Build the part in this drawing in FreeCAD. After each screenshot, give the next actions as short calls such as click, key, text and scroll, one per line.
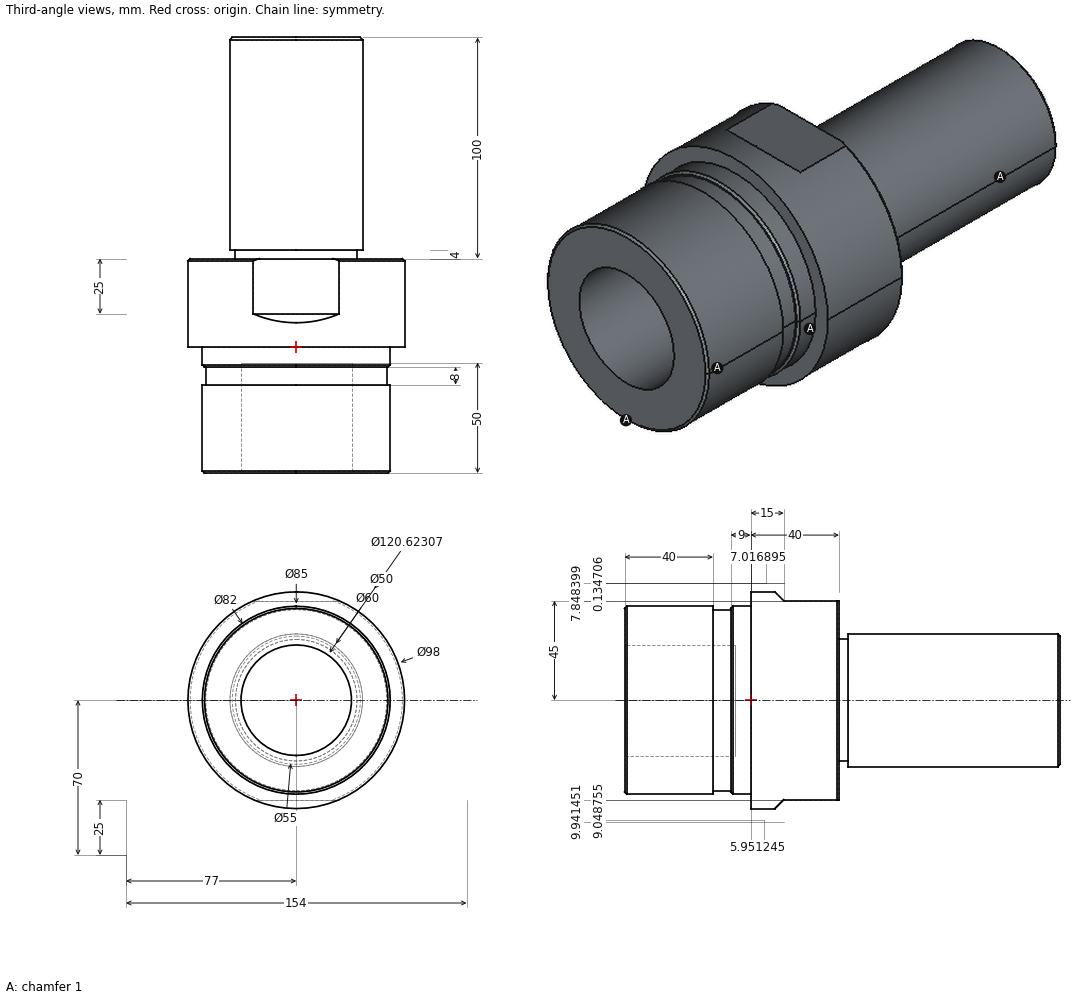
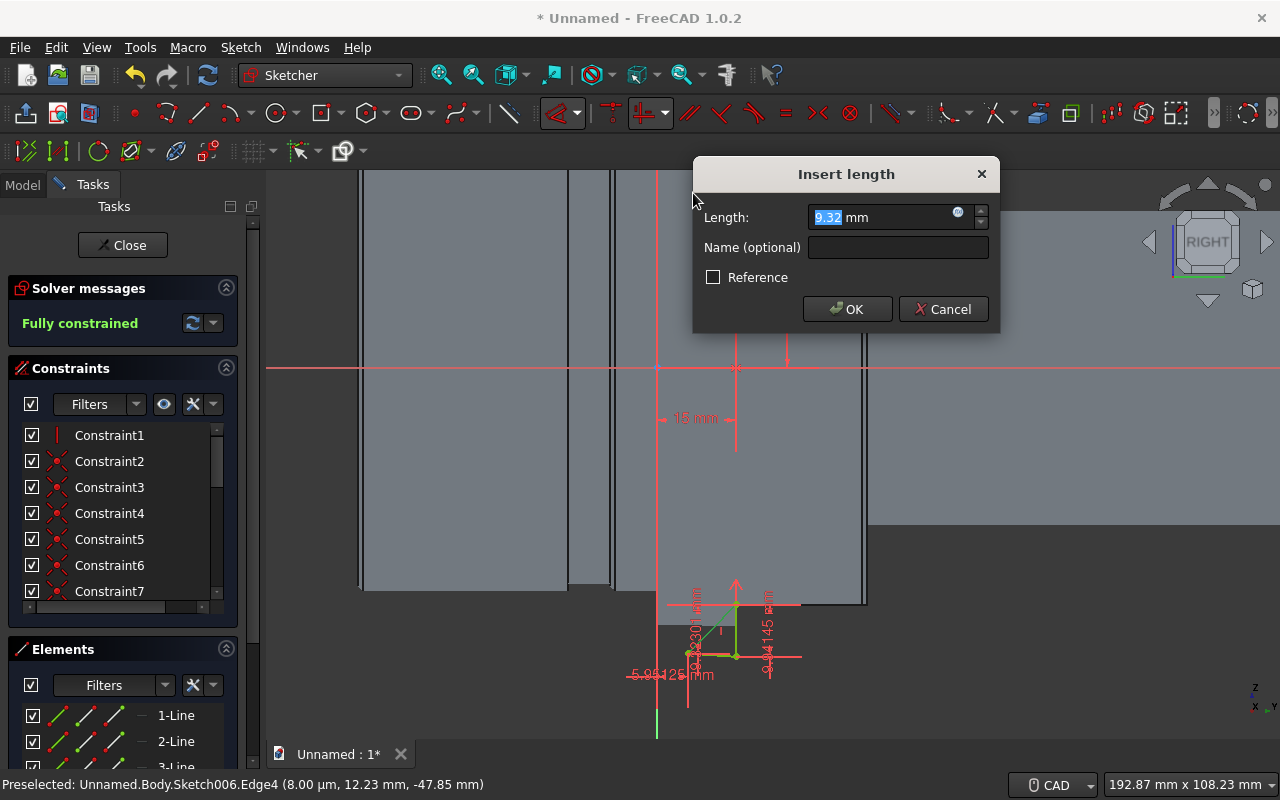
text(9.048755)
key(Return)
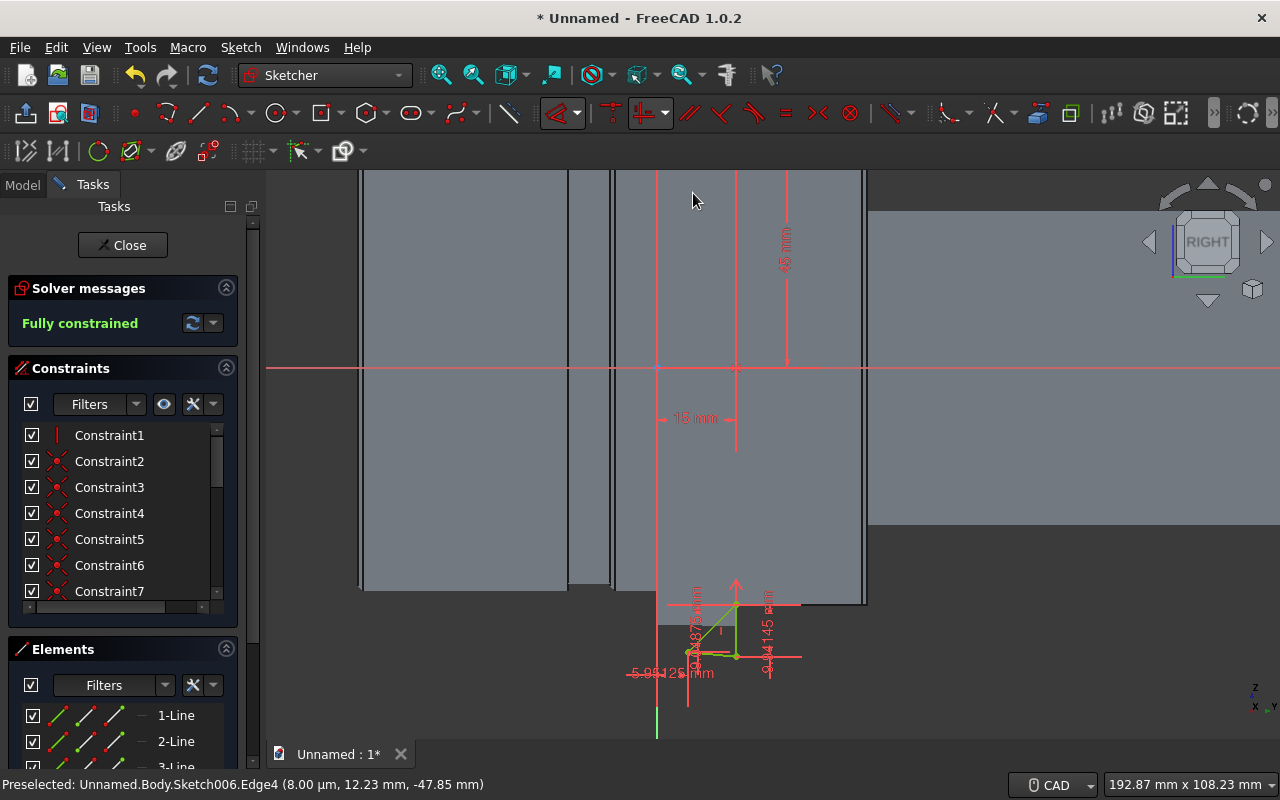
click(123, 245)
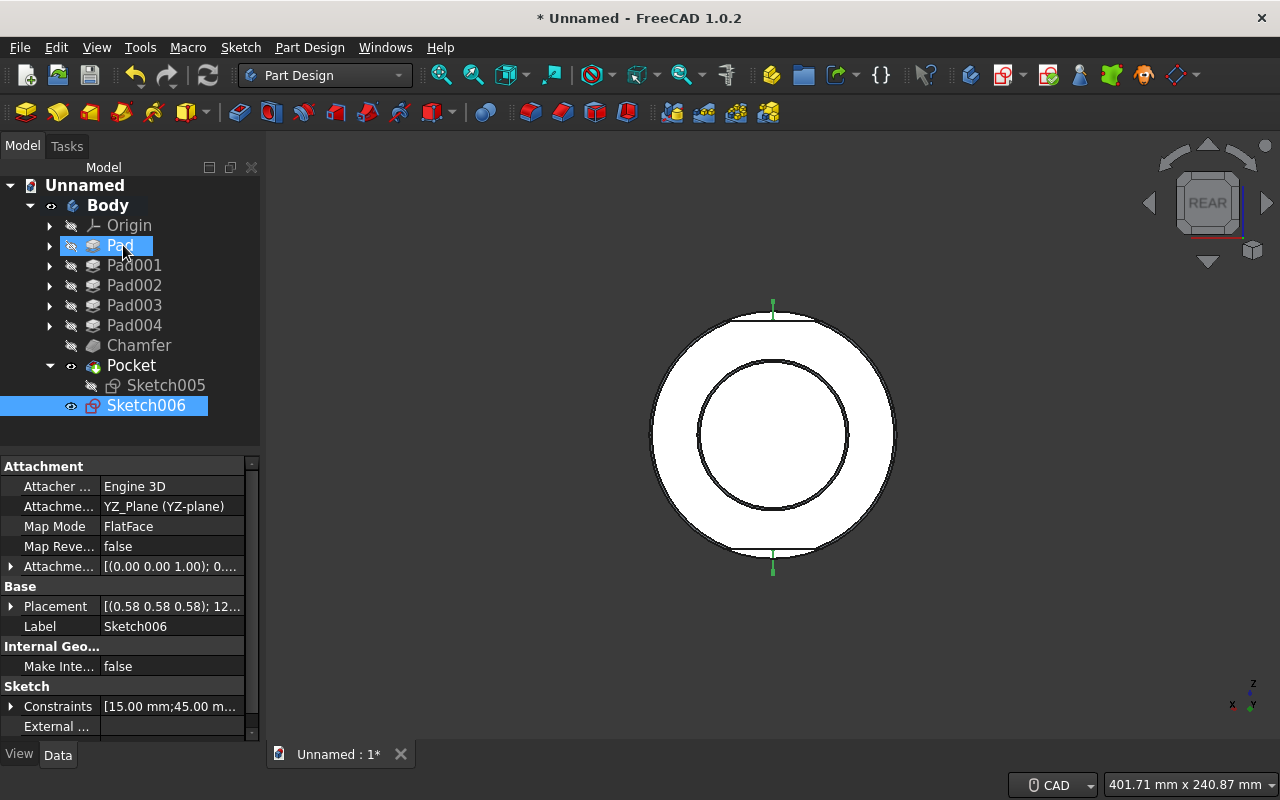
click(240, 112)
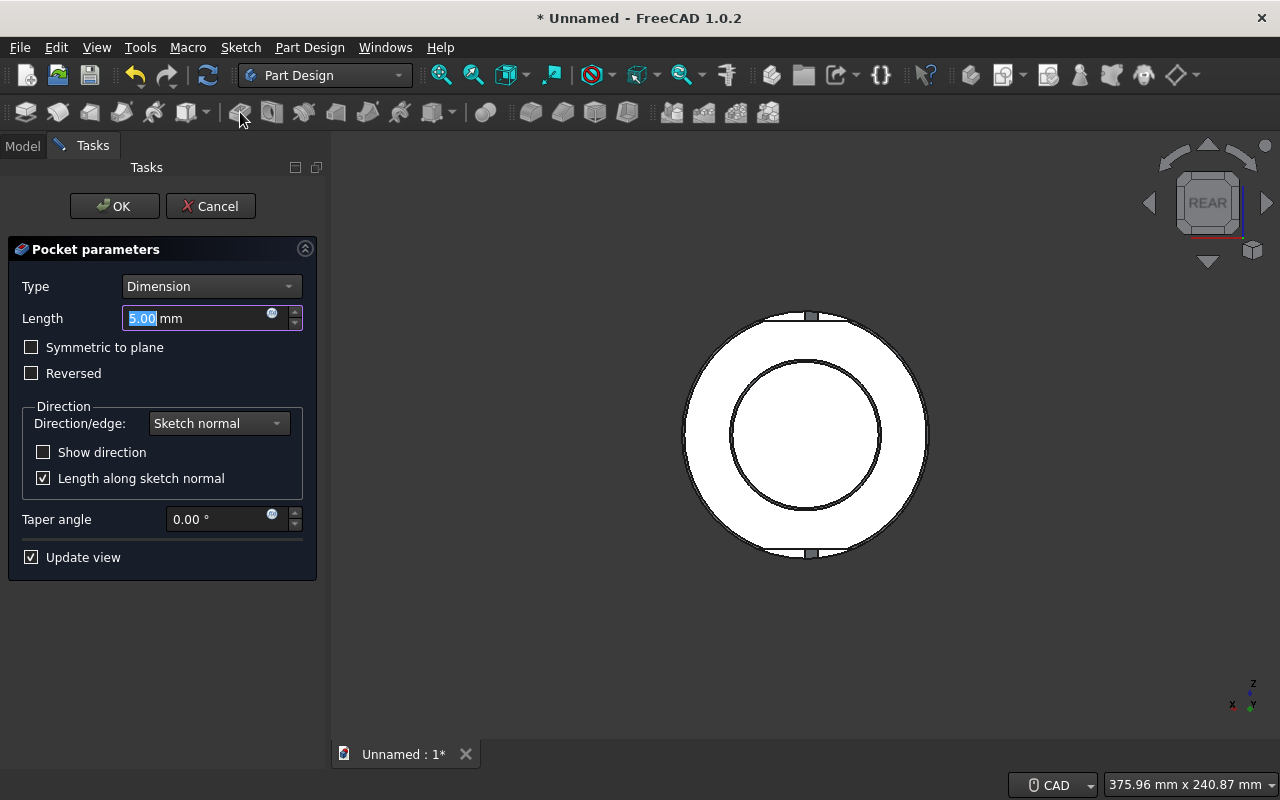
click(212, 286)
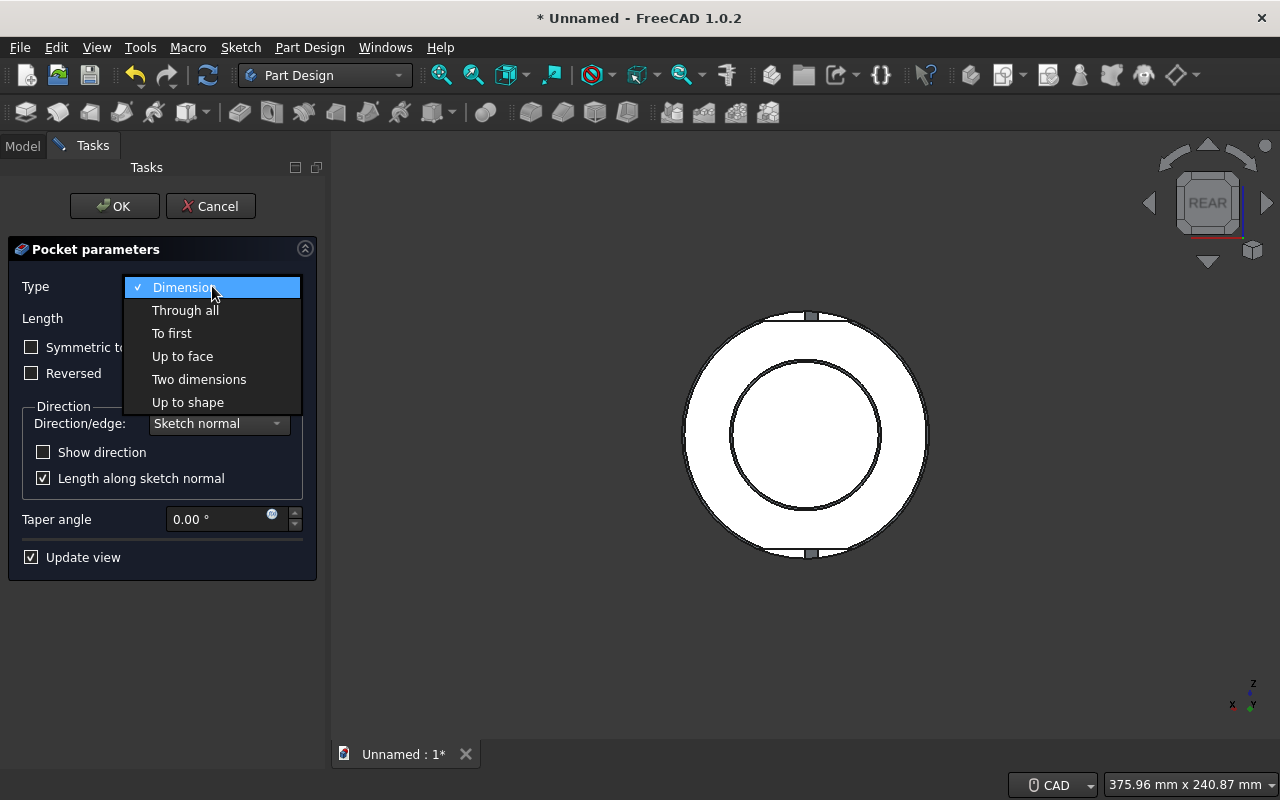
click(212, 310)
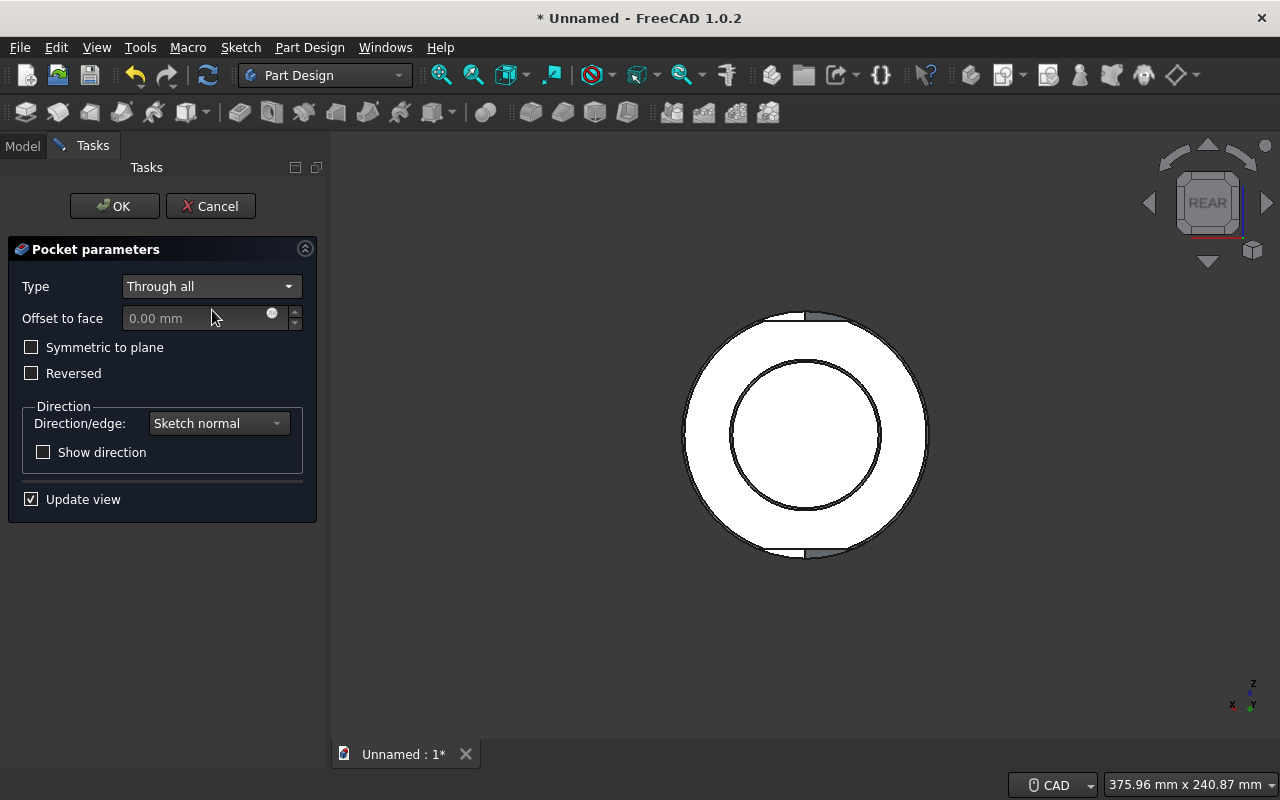
click(115, 206)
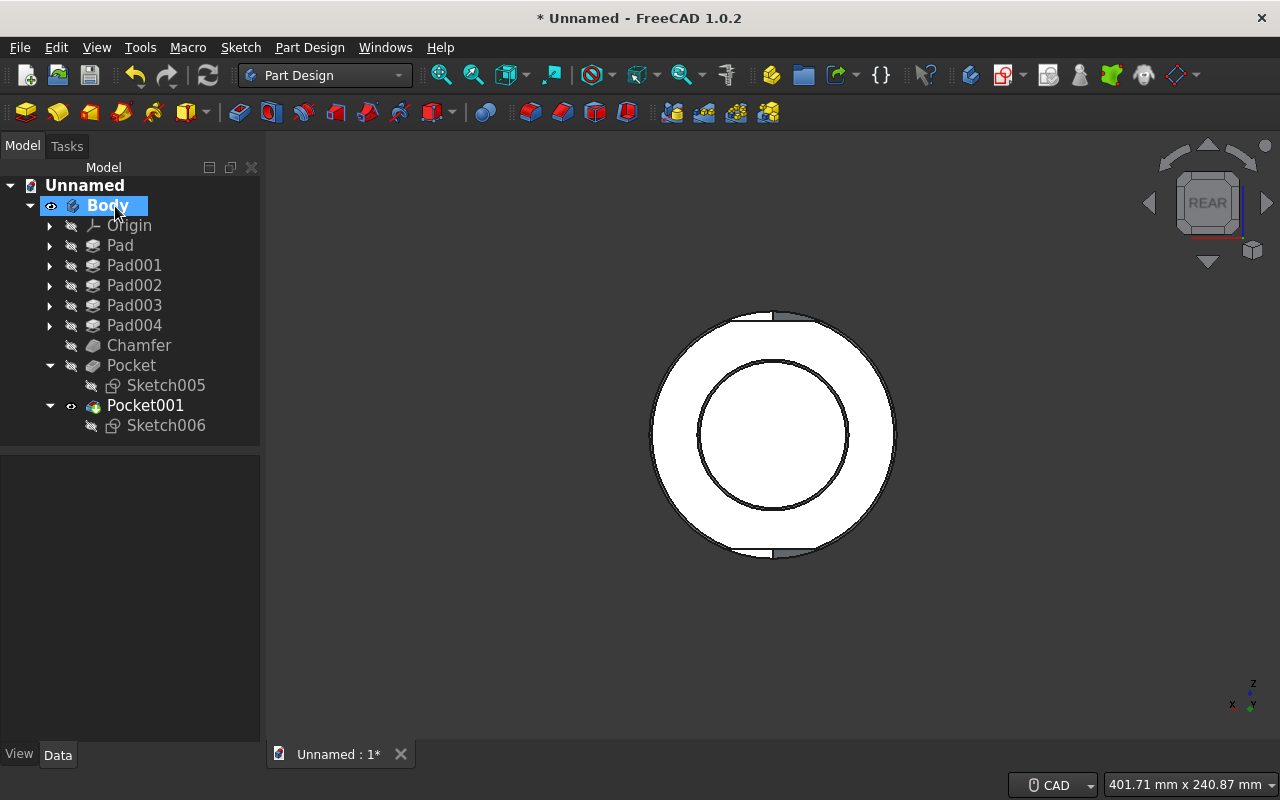
click(442, 76)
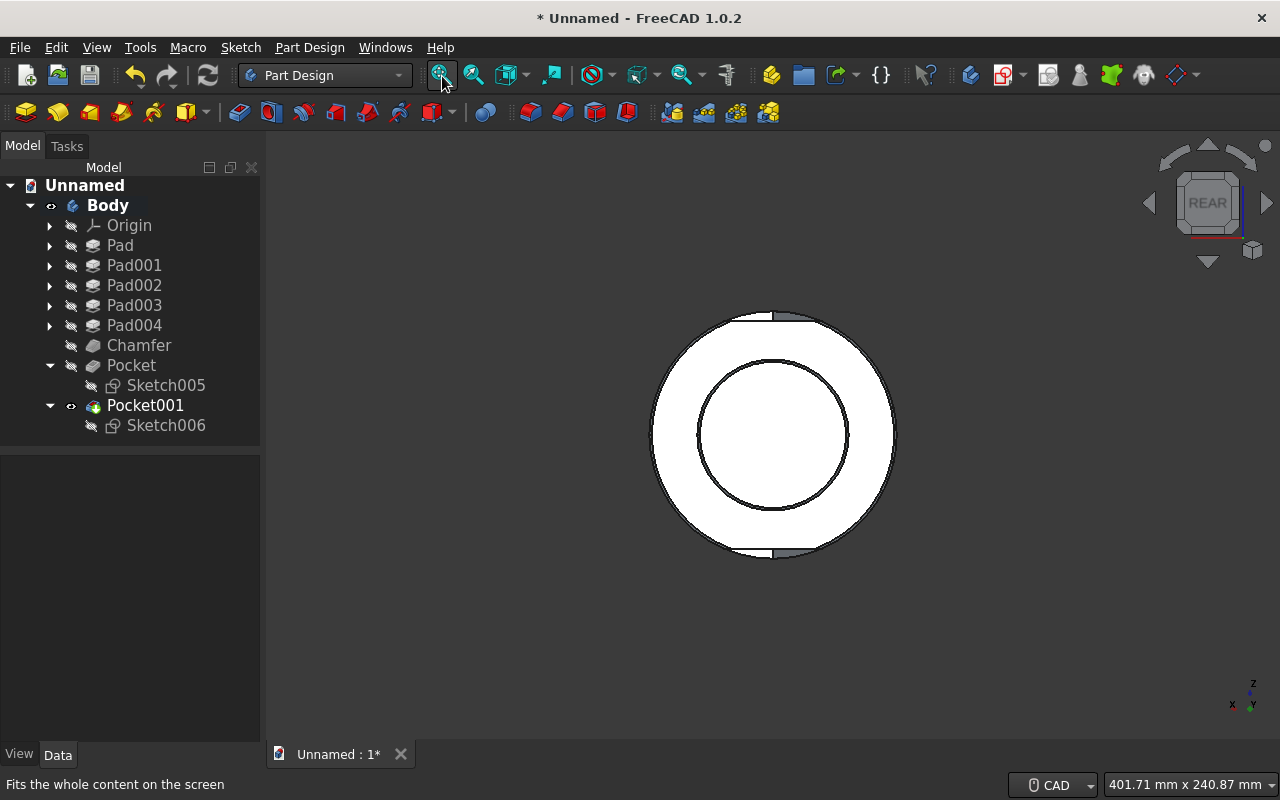
click(1004, 76)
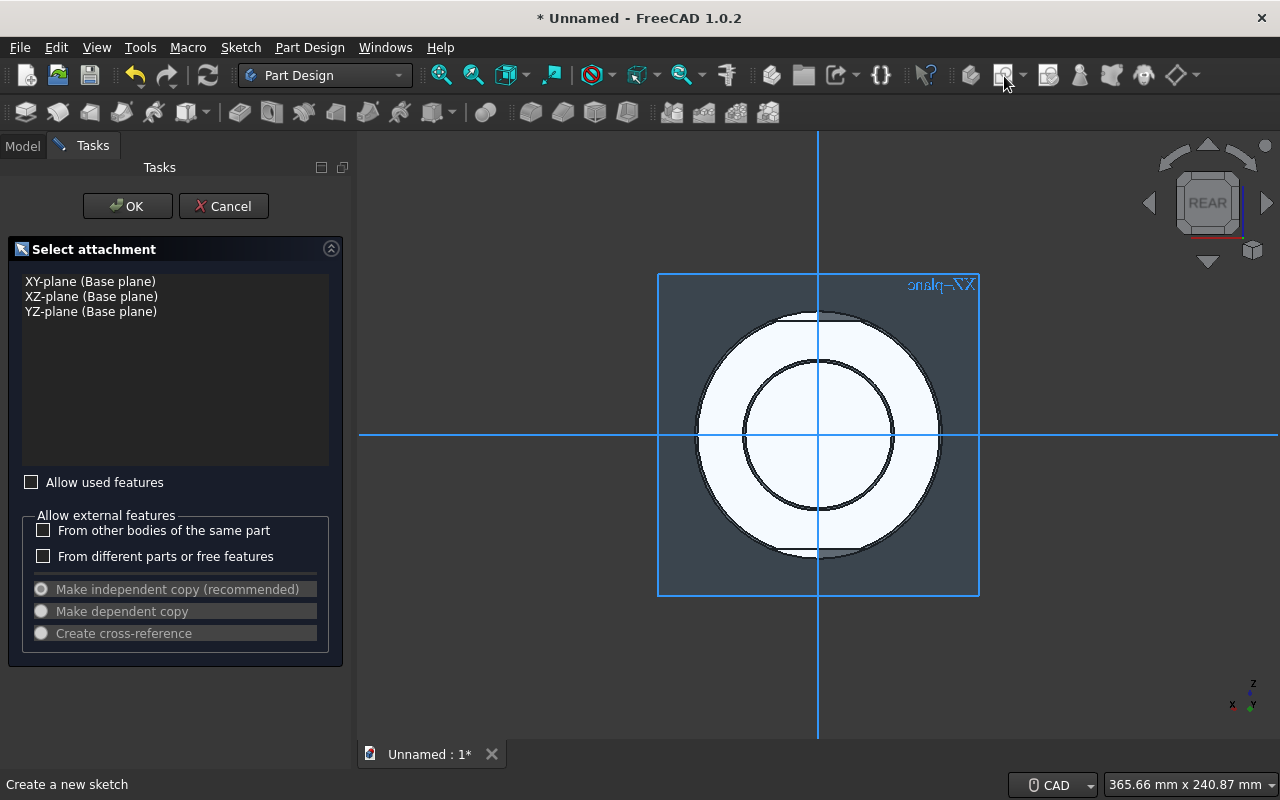
click(82, 312)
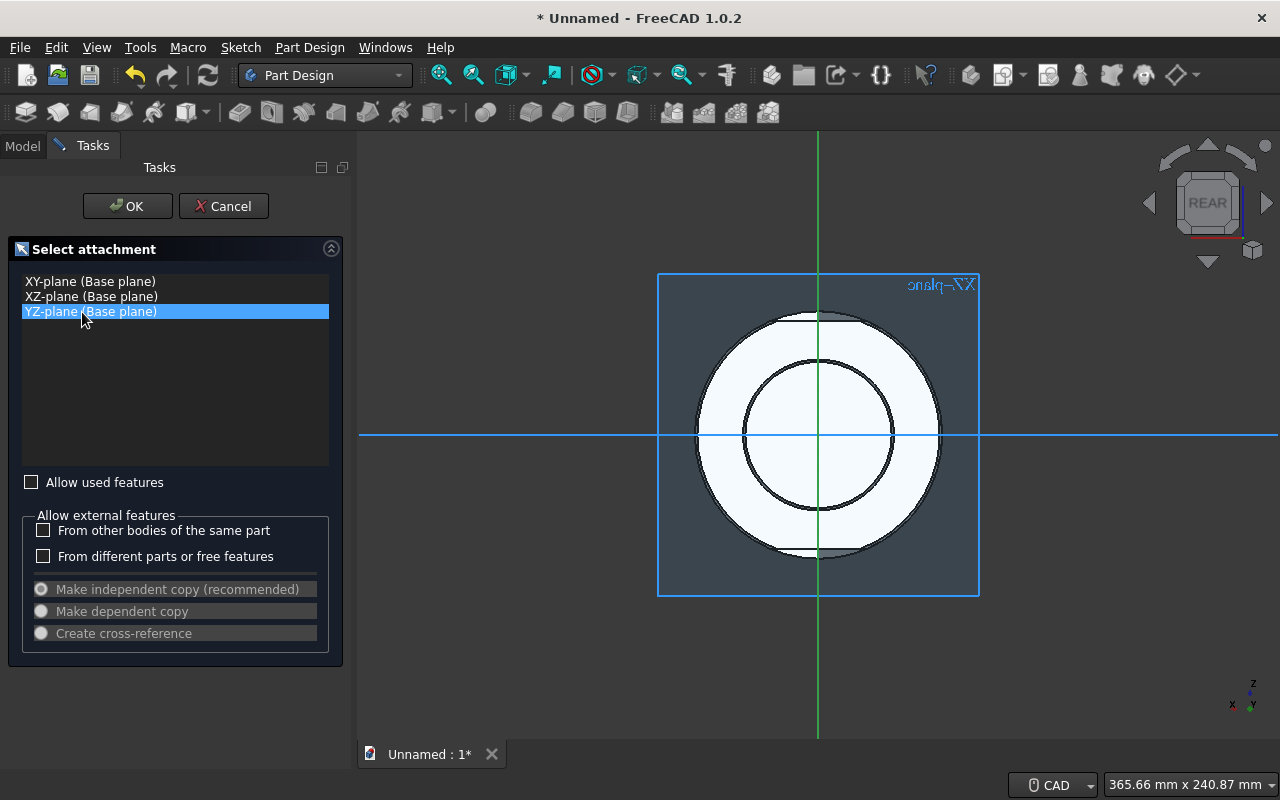
click(128, 206)